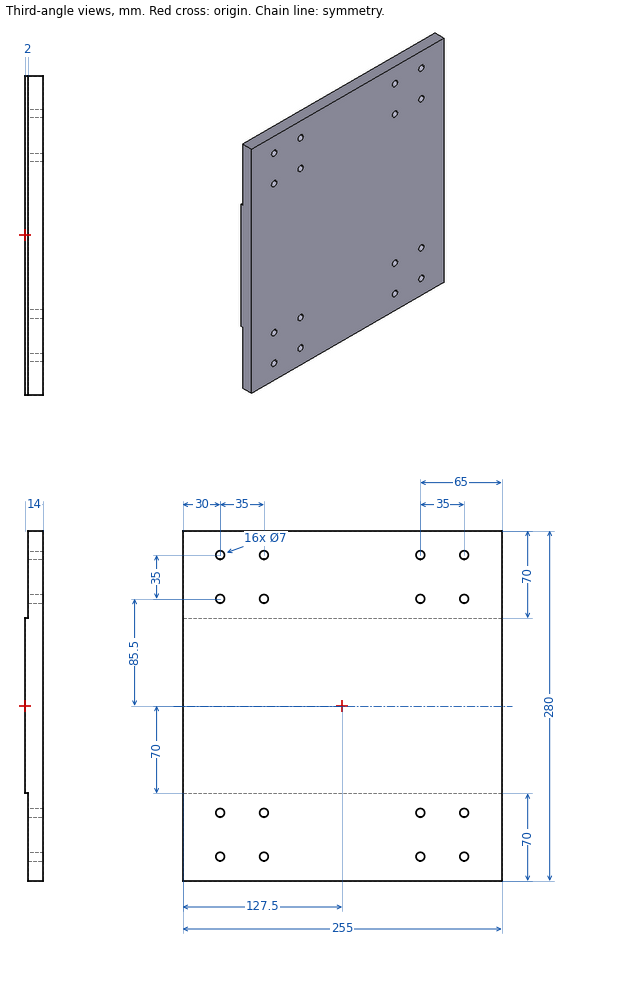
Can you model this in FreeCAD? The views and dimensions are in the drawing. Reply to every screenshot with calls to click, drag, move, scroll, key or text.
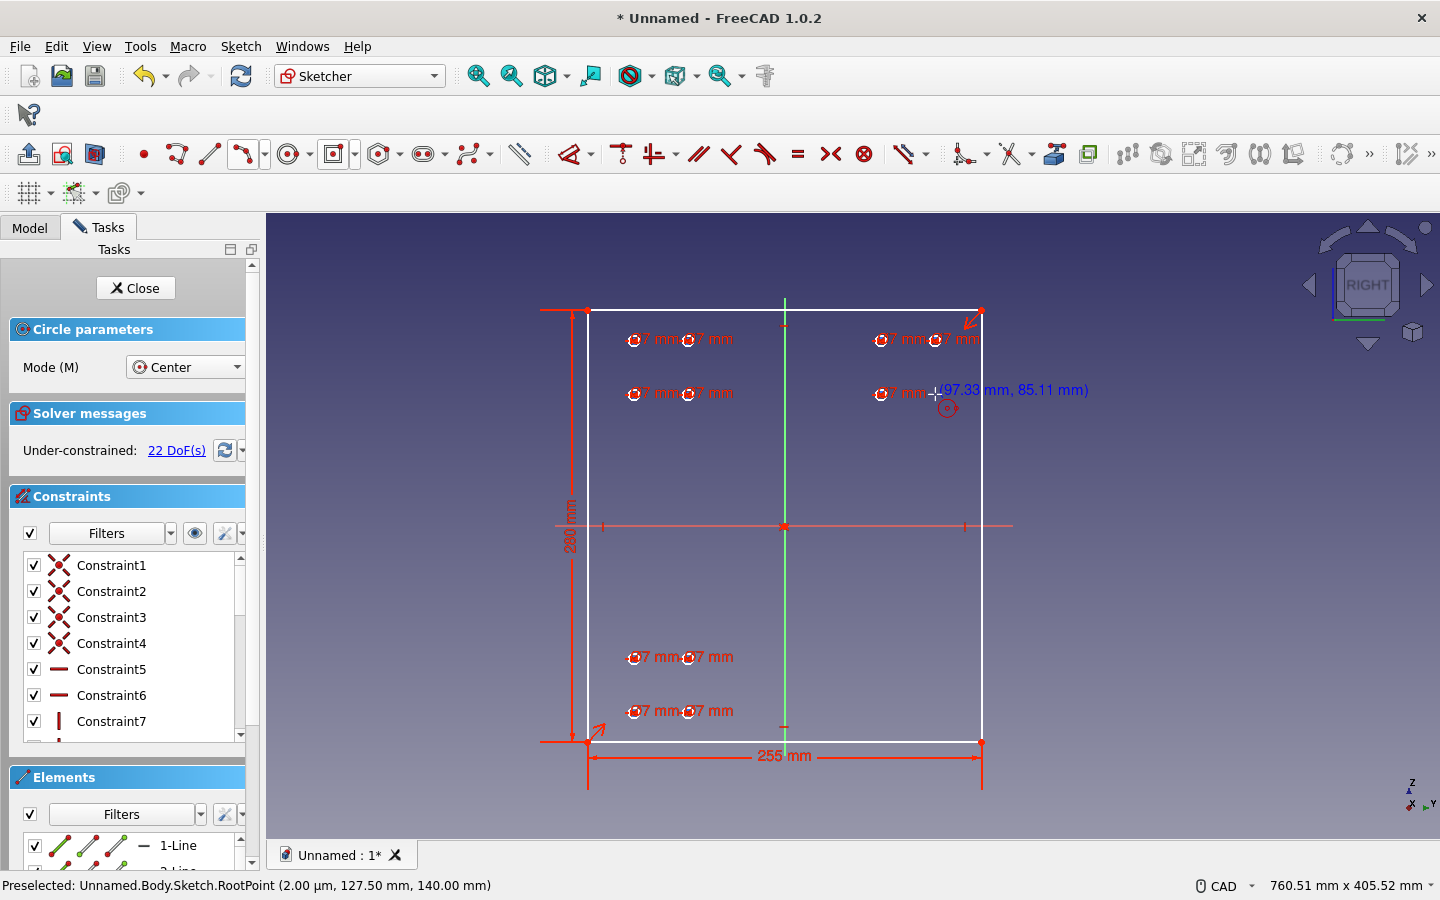
click(935, 394)
move(939, 391)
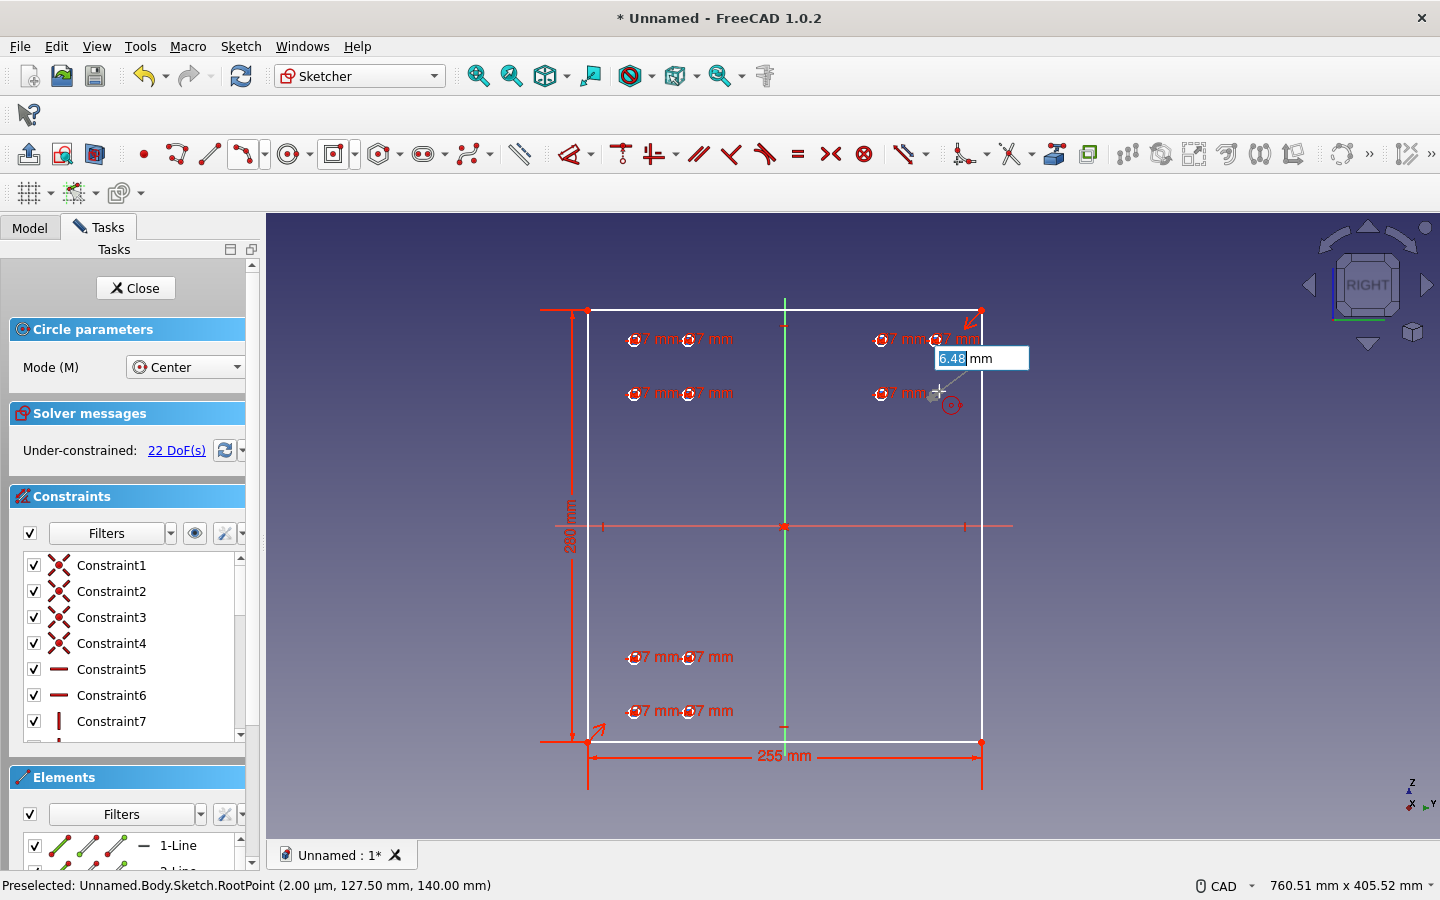
text(7)
key(Return)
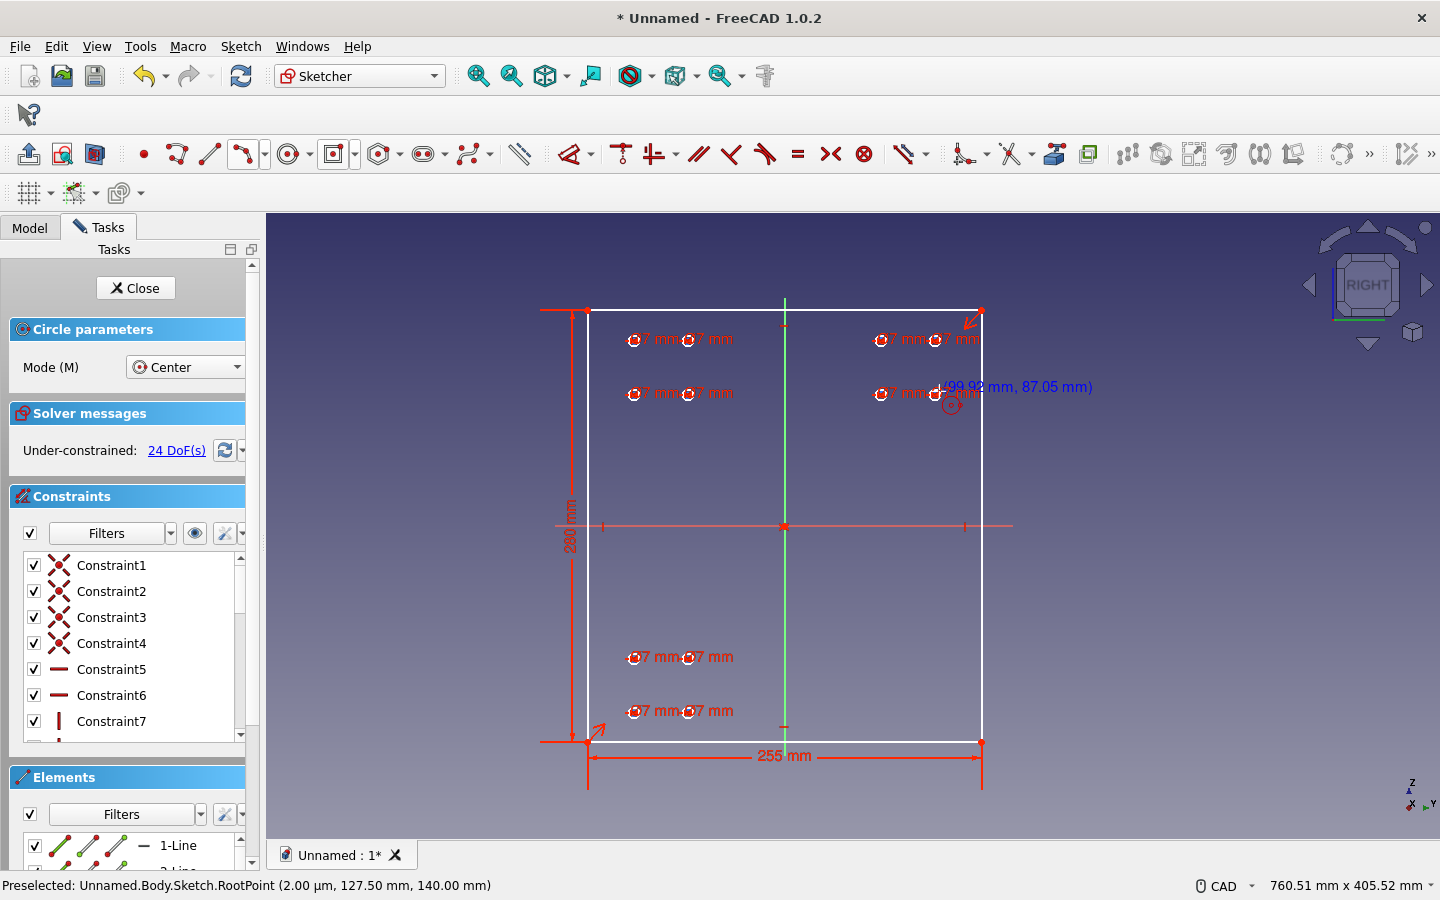
scroll(881, 658, up, 8)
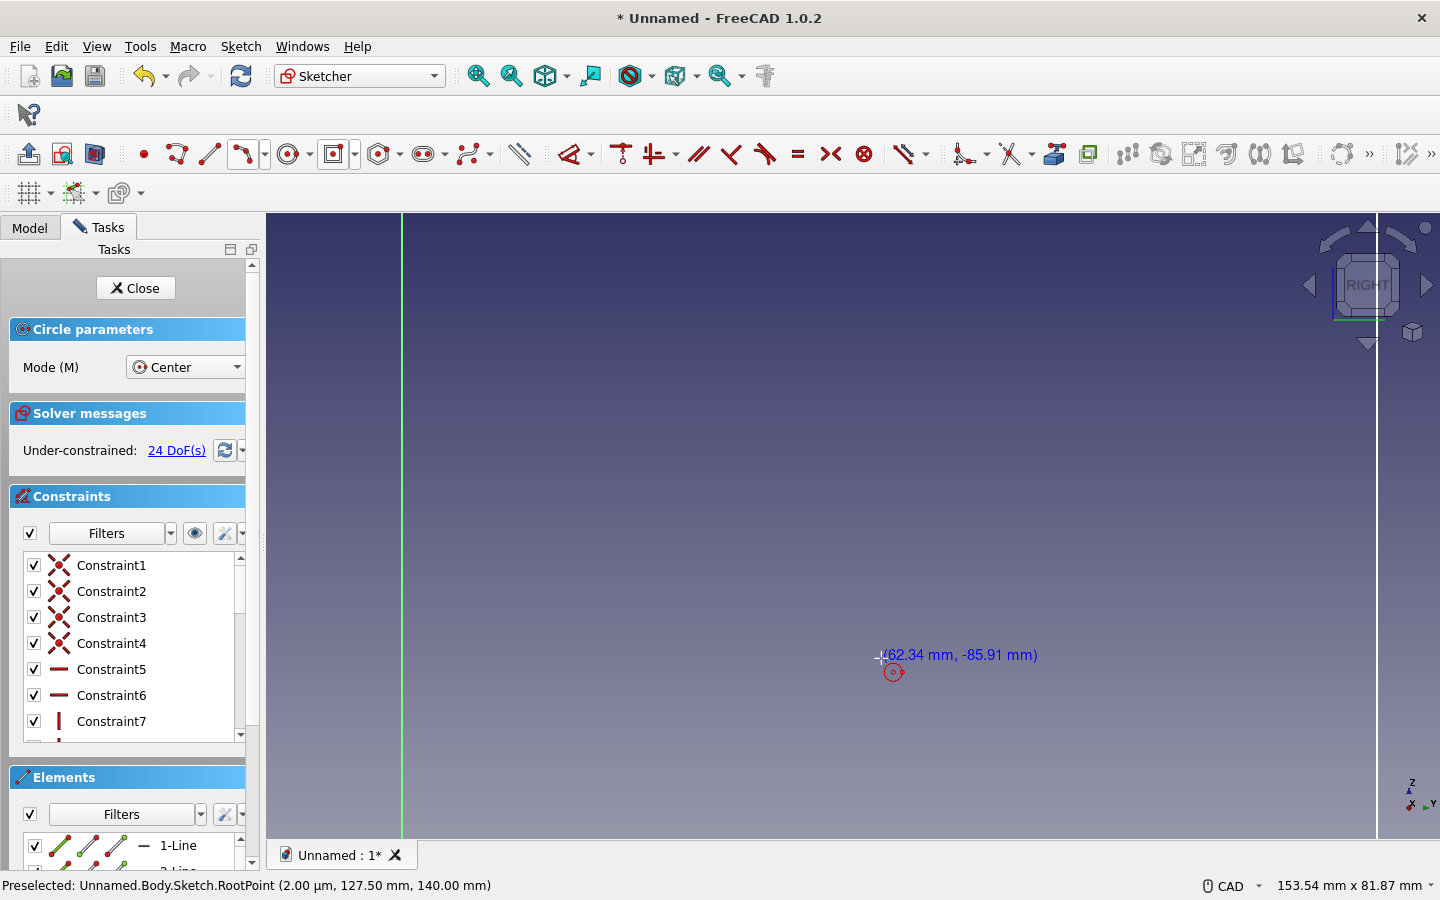
scroll(881, 658, down, 8)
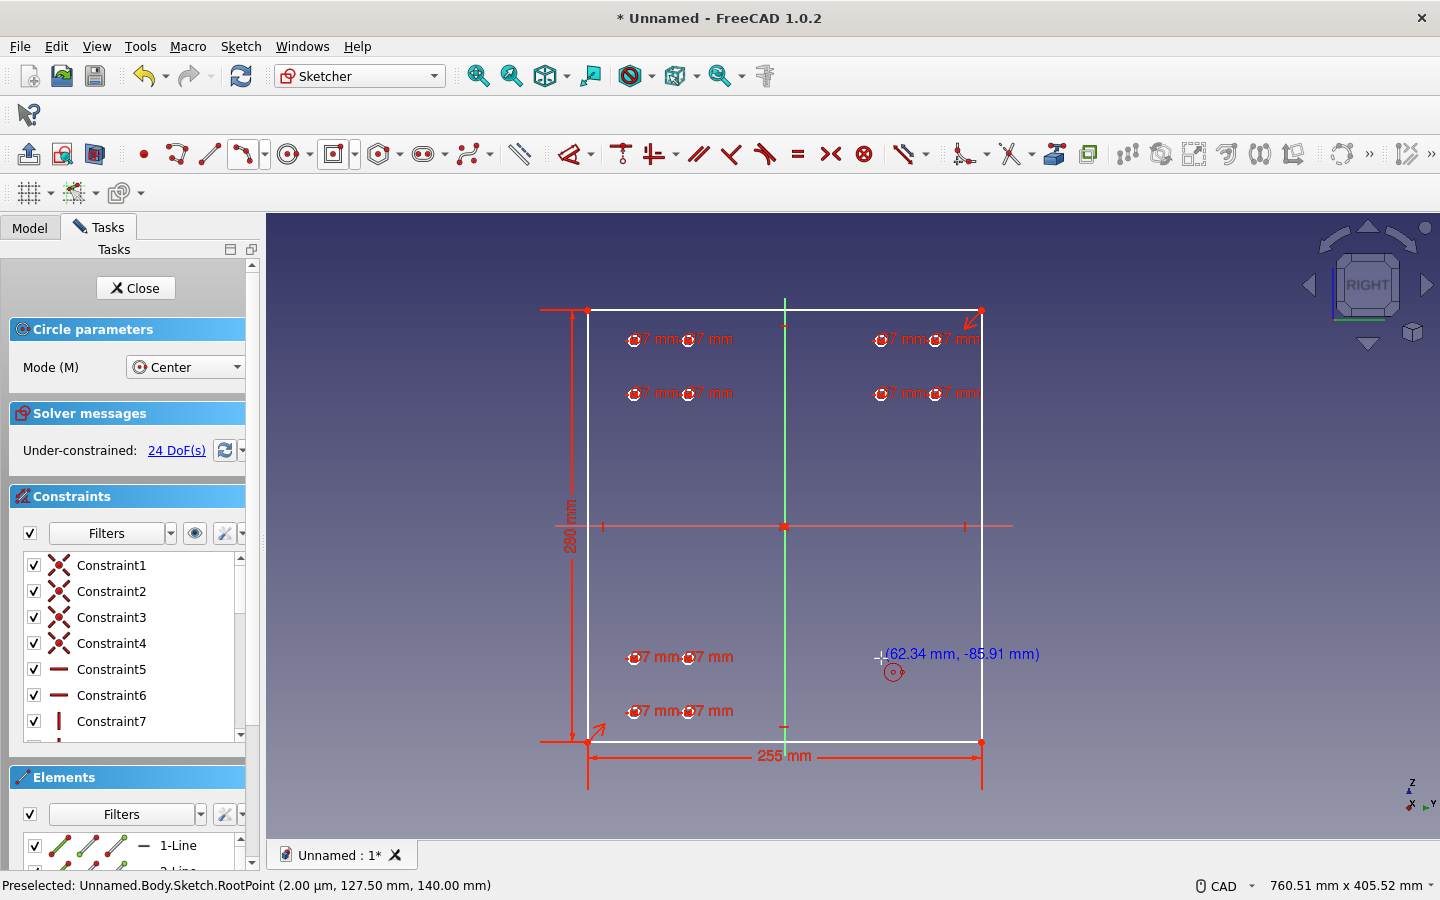
click(881, 658)
move(885, 655)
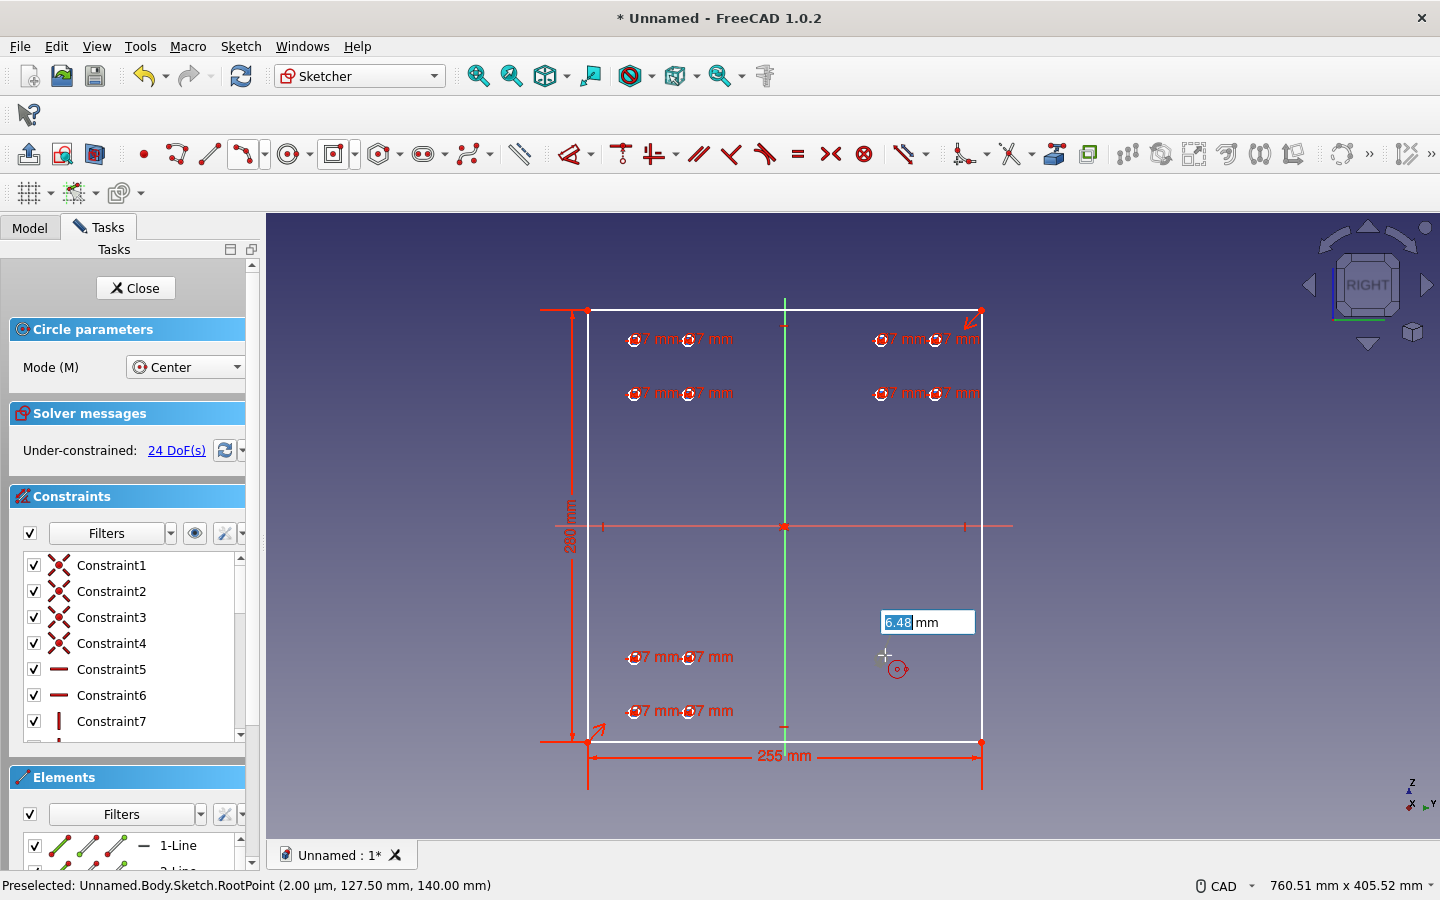
text(7)
key(Return)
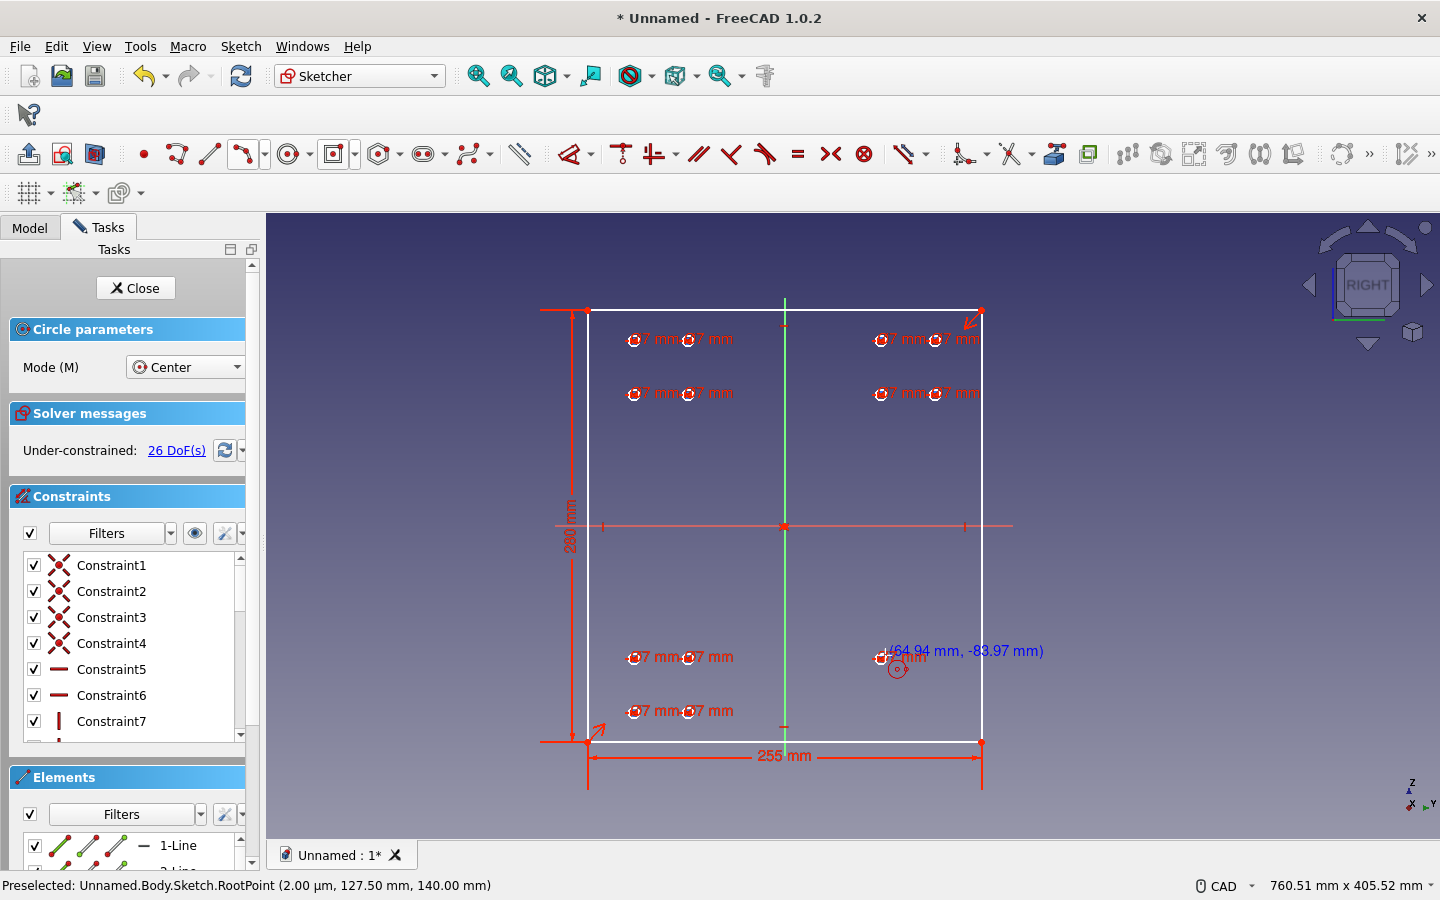
scroll(881, 712, up, 8)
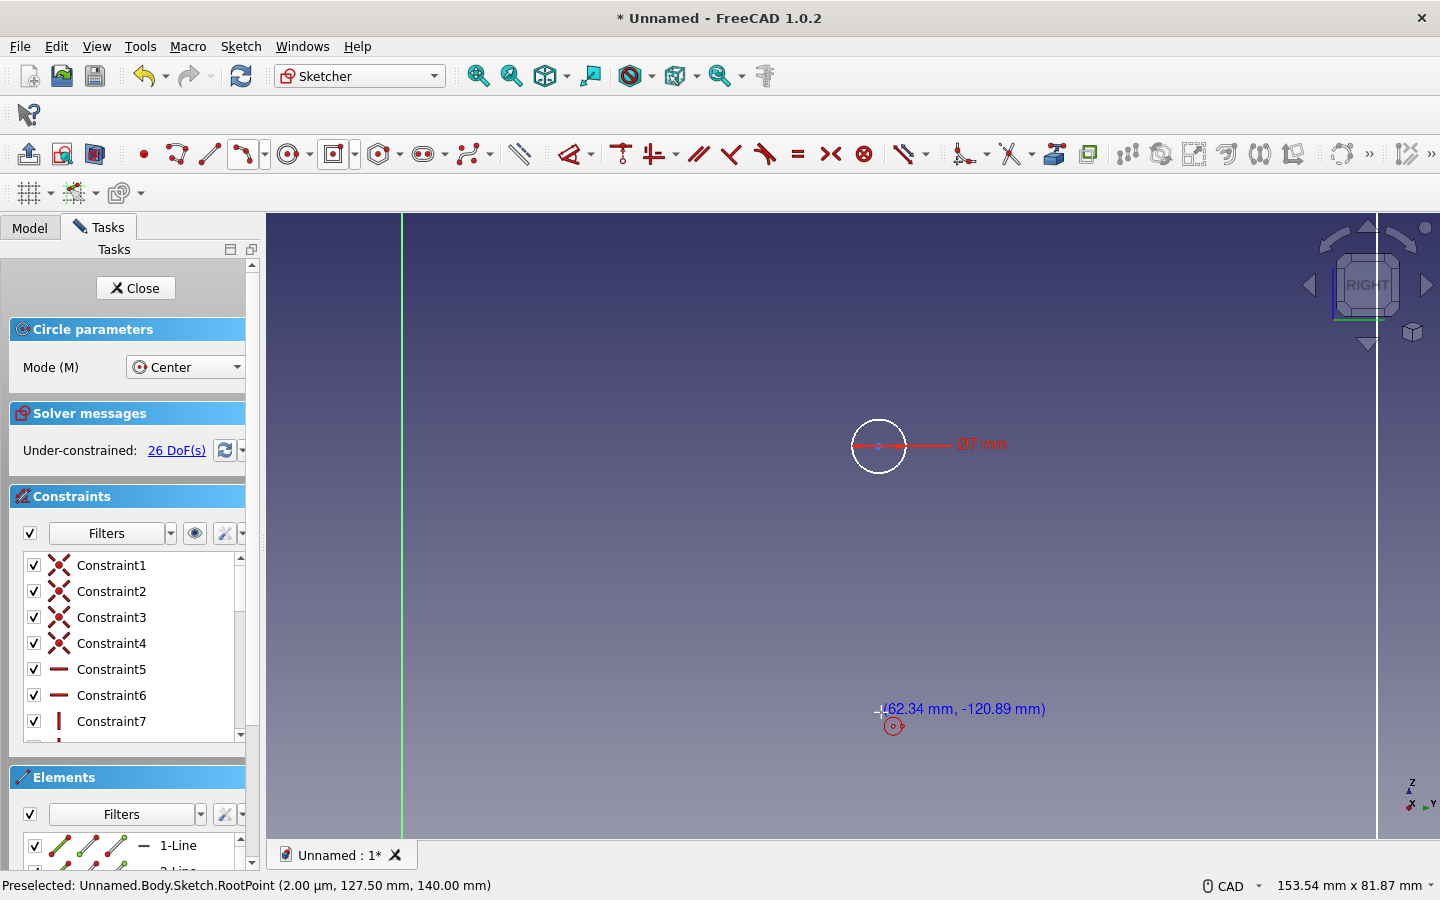
scroll(881, 712, down, 8)